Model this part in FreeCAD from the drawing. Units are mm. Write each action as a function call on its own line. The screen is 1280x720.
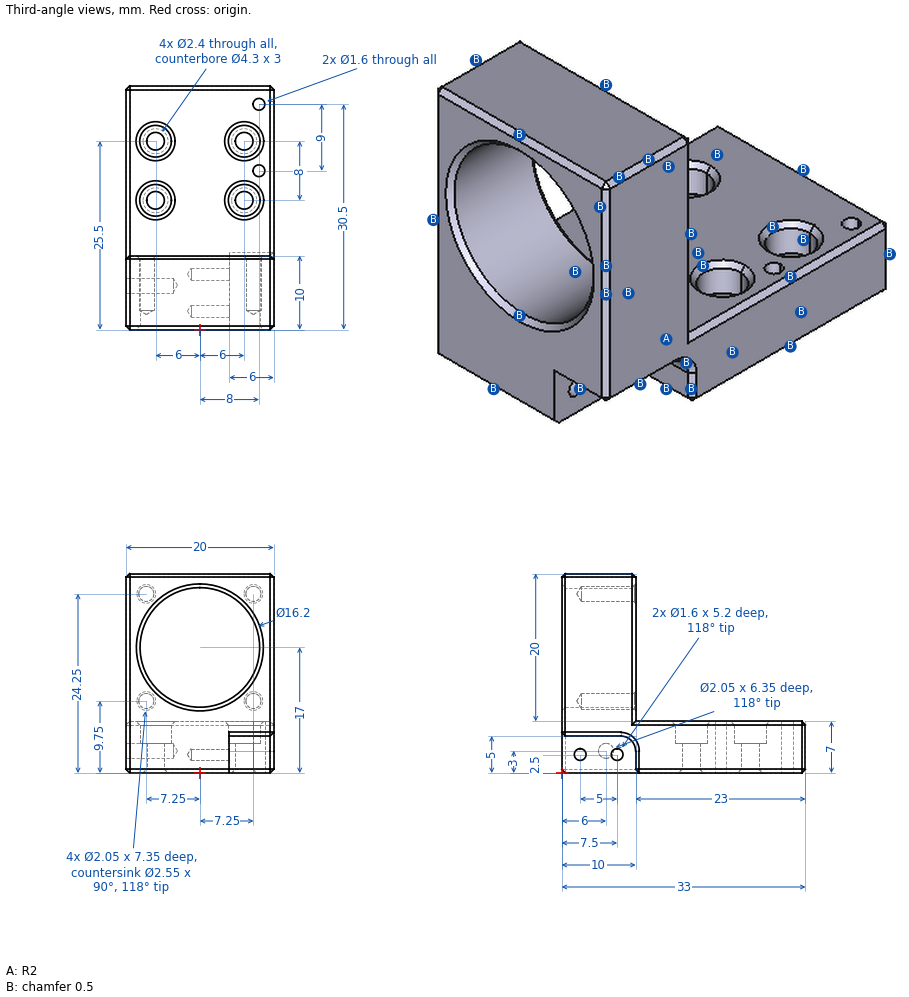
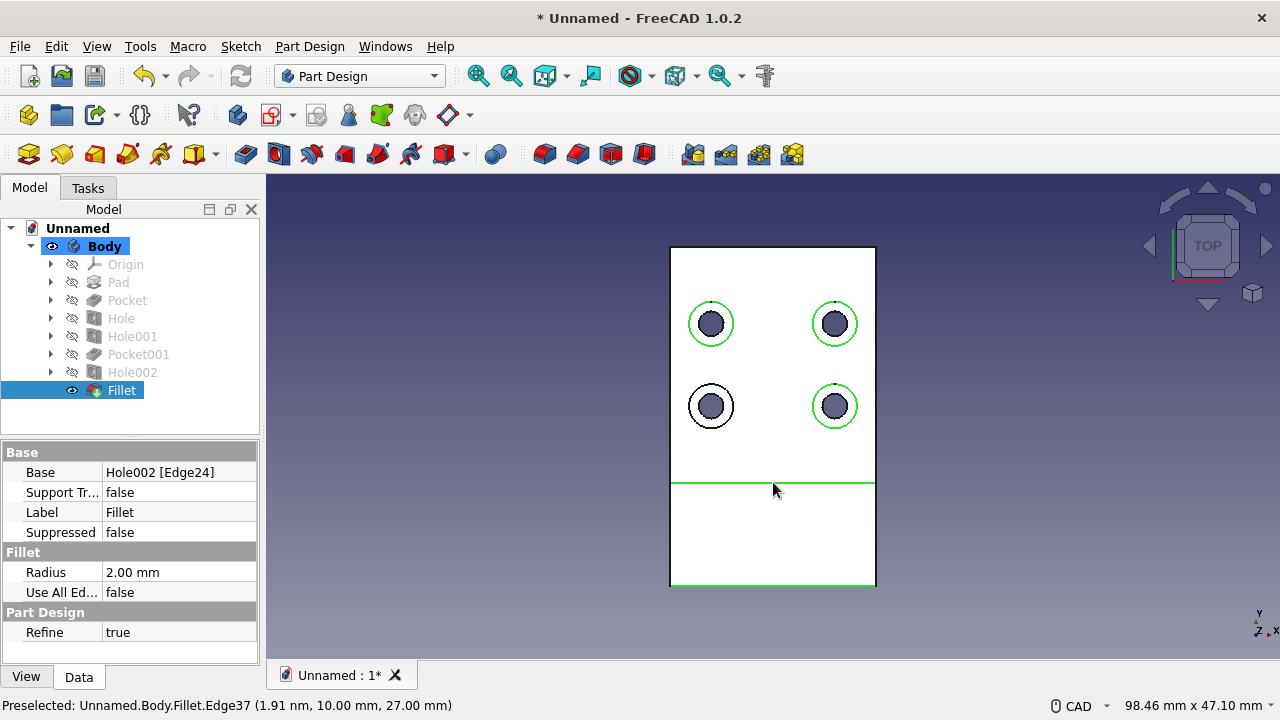
click(773, 246, ctrl)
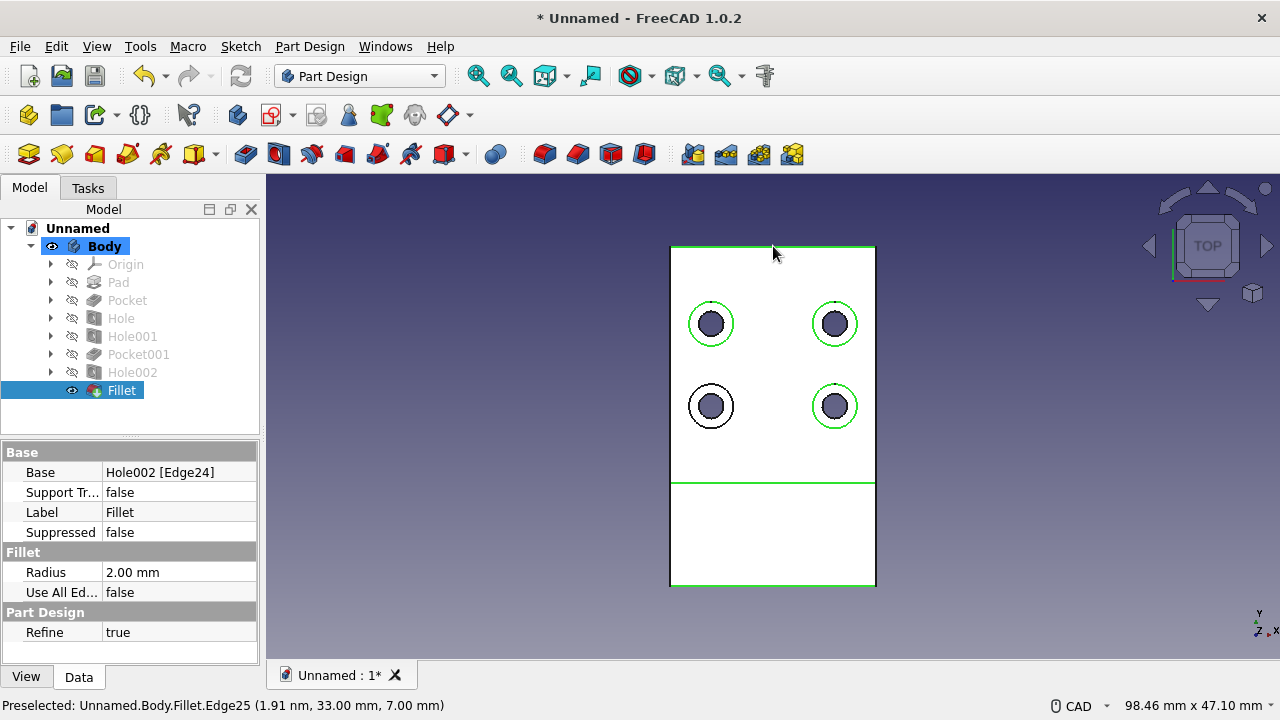
click(711, 427, ctrl)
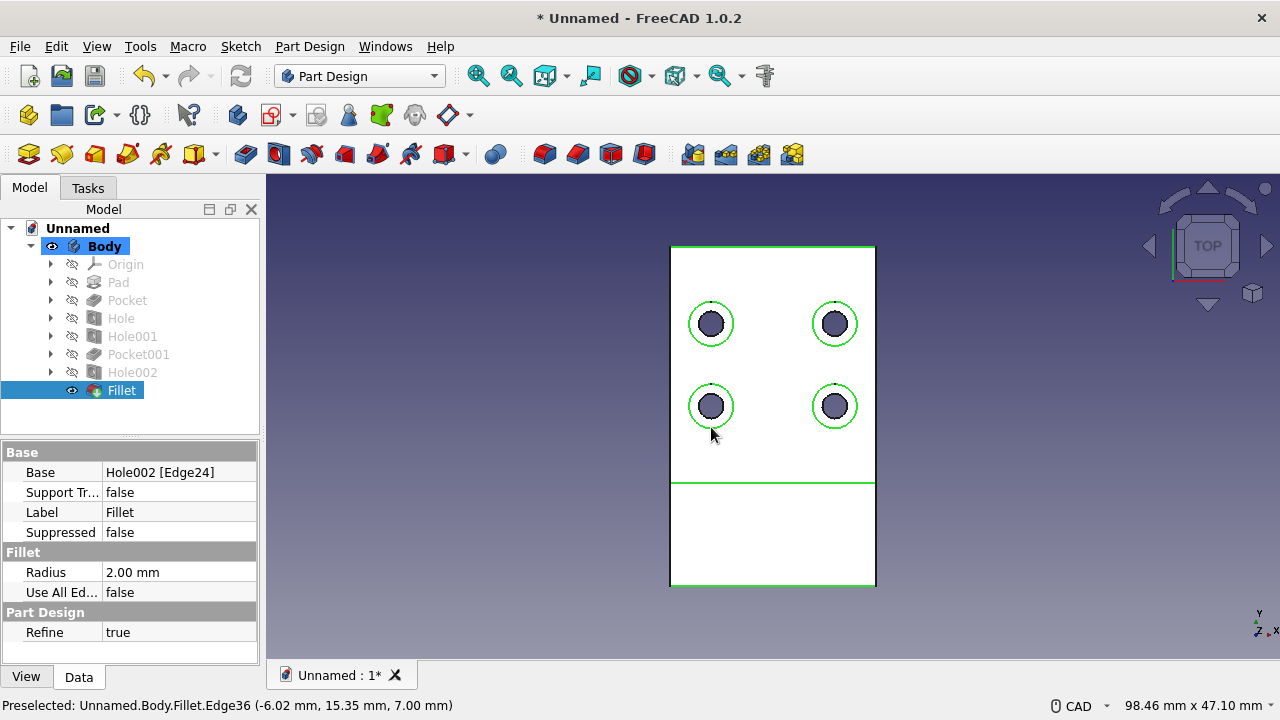
key(0)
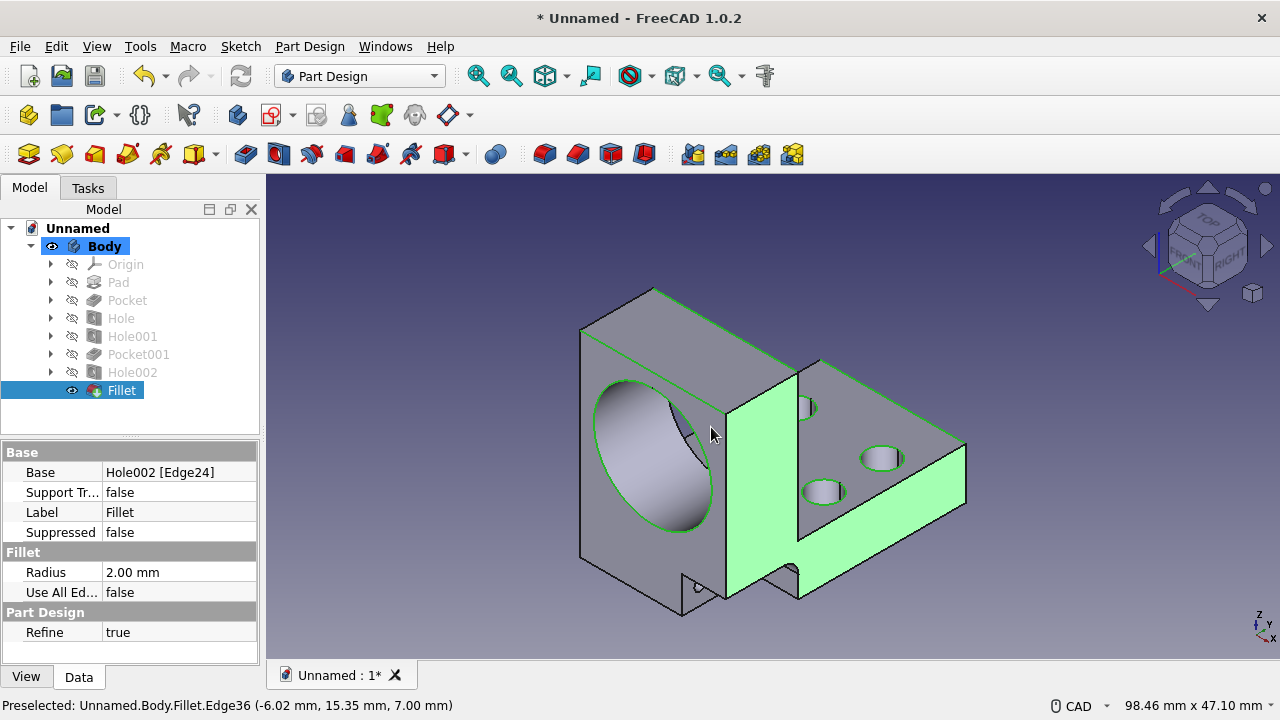
key(1)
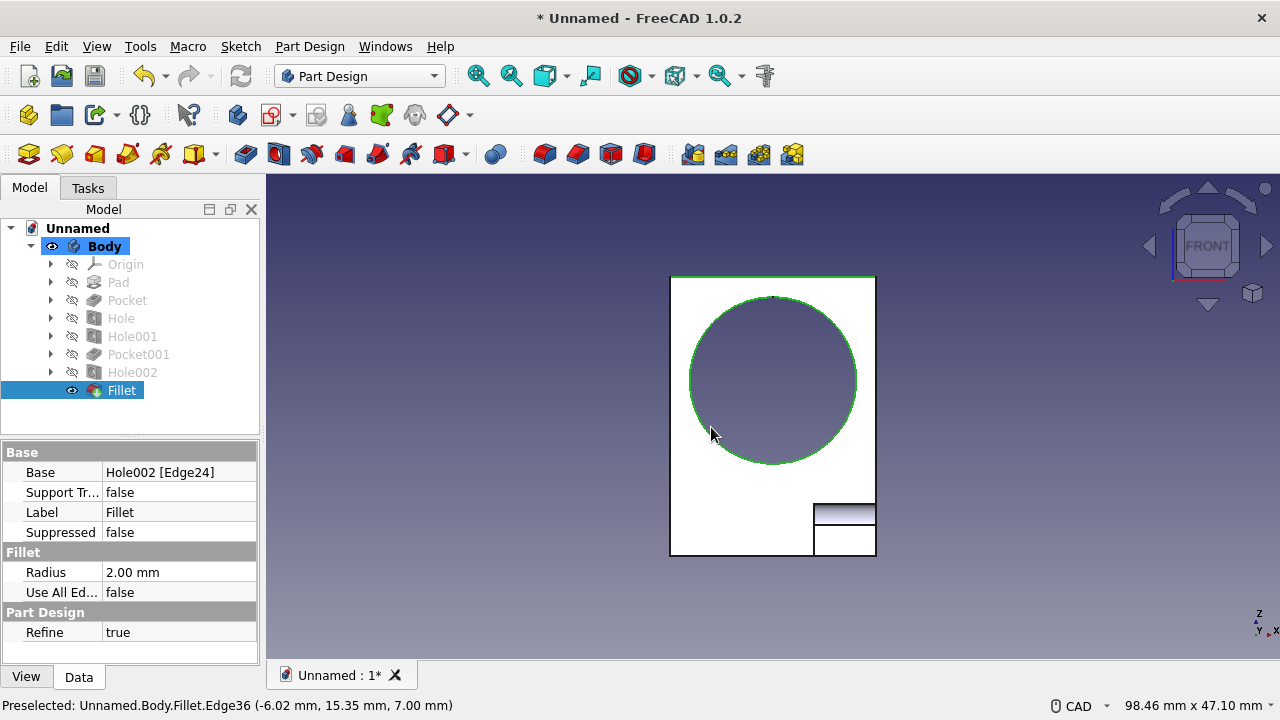
click(742, 555, ctrl)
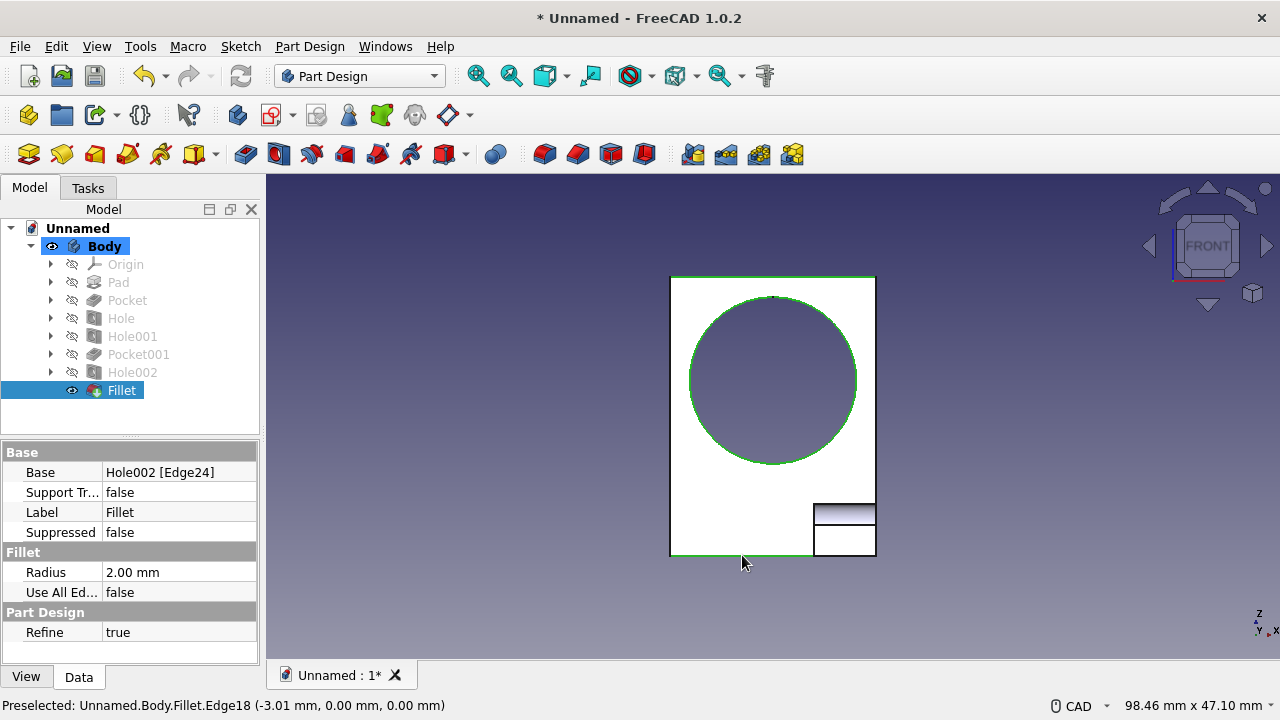
click(845, 555, ctrl)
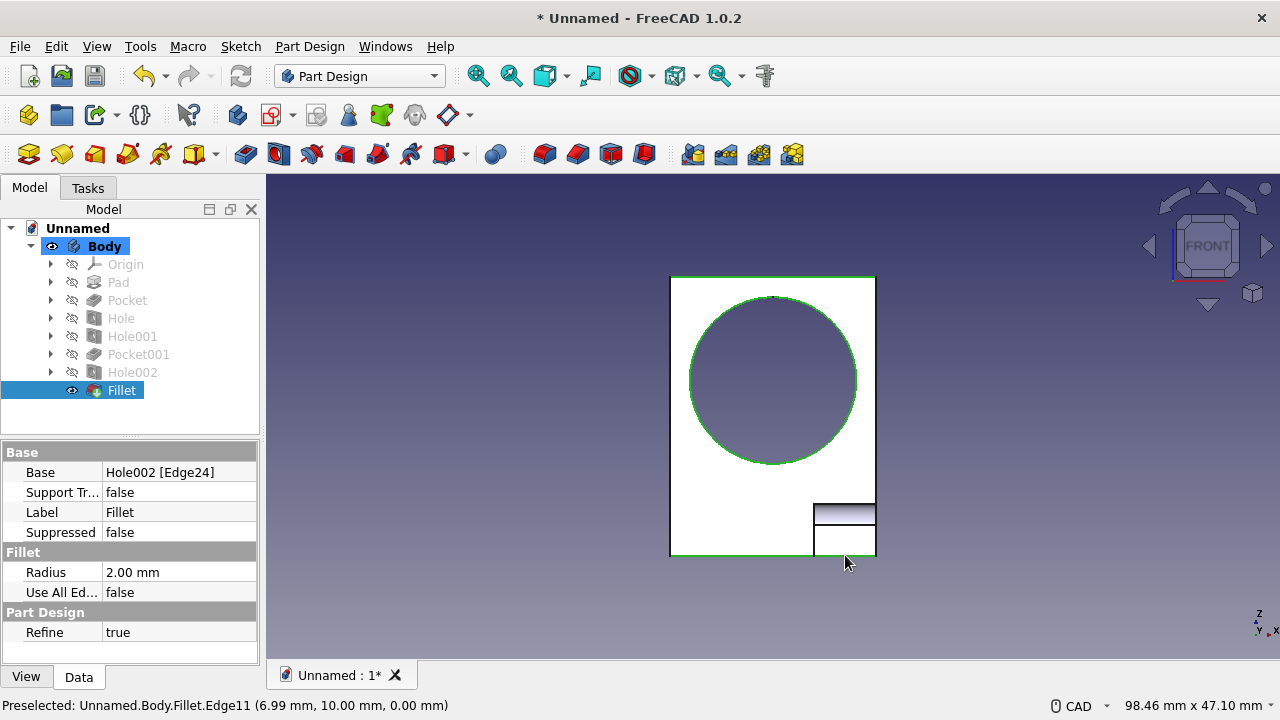
click(845, 503, ctrl)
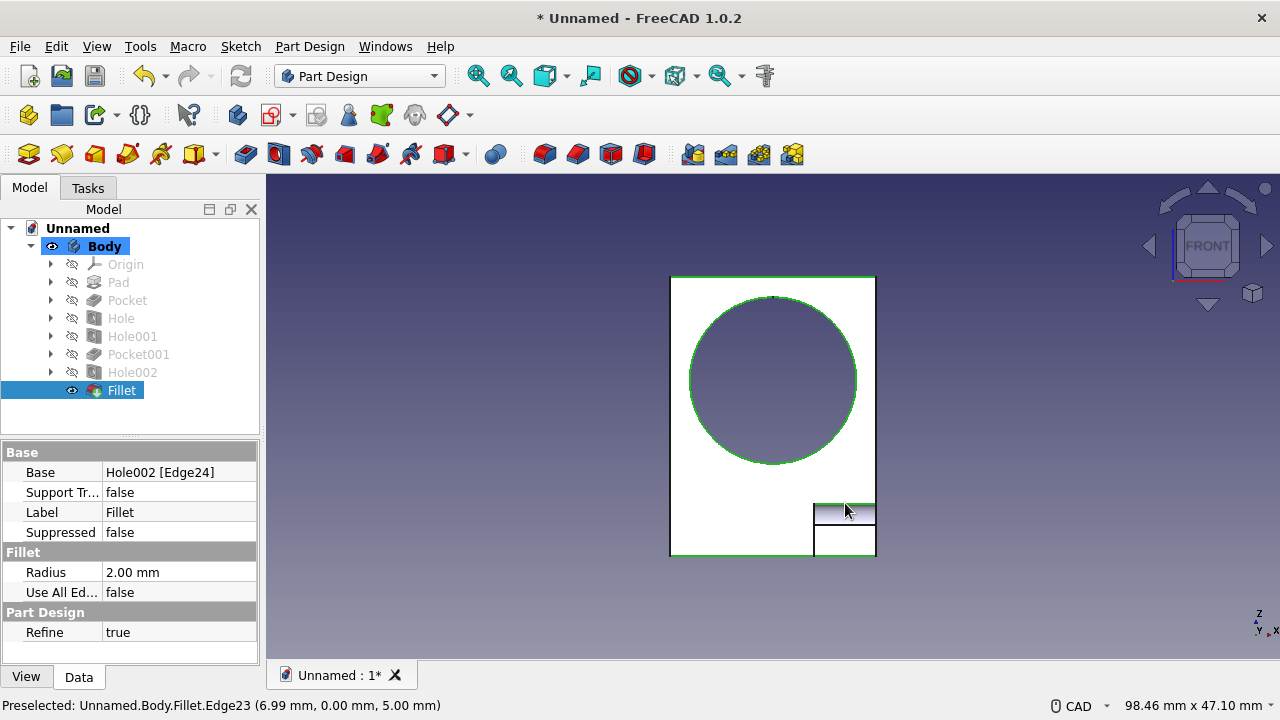
key(3)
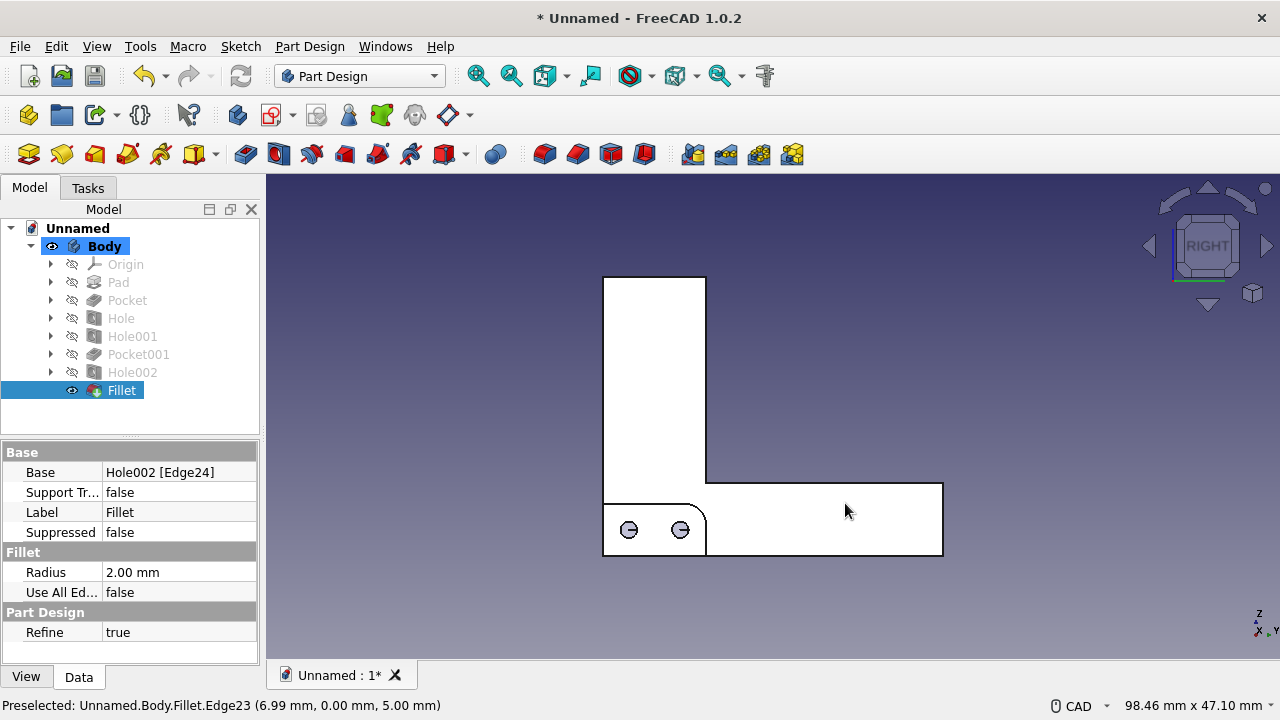
key(5)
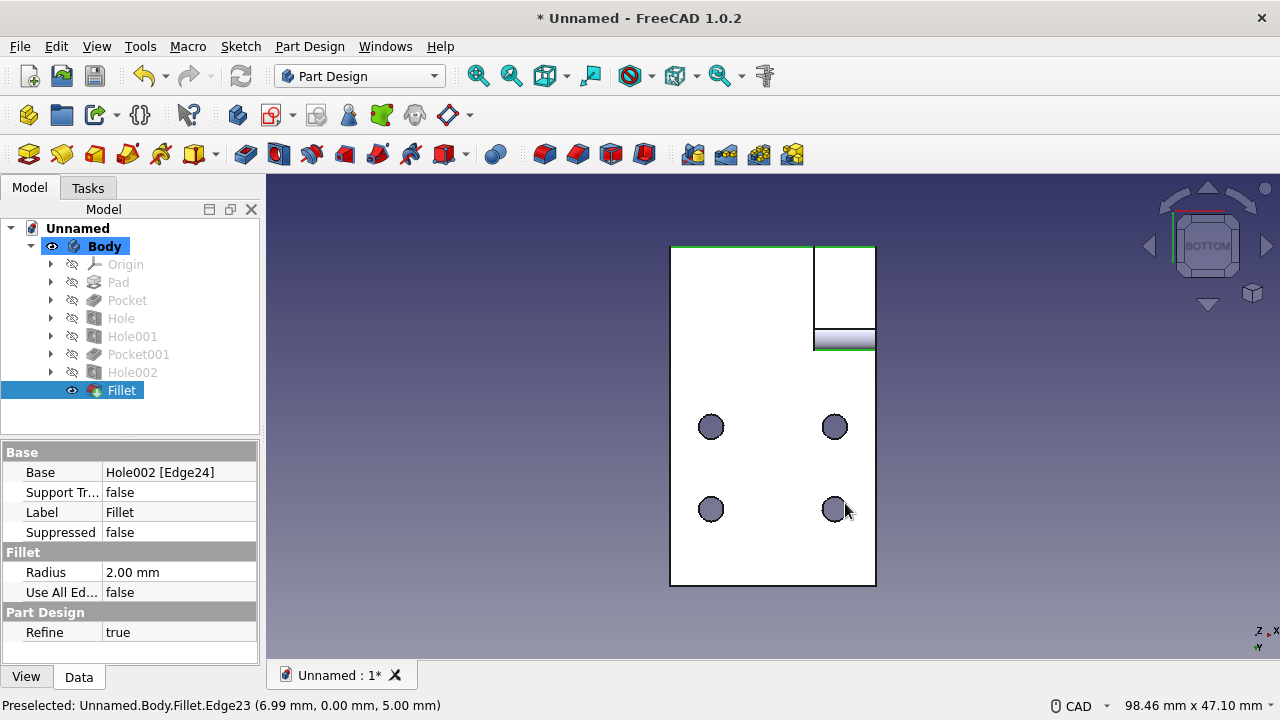
click(773, 585, ctrl)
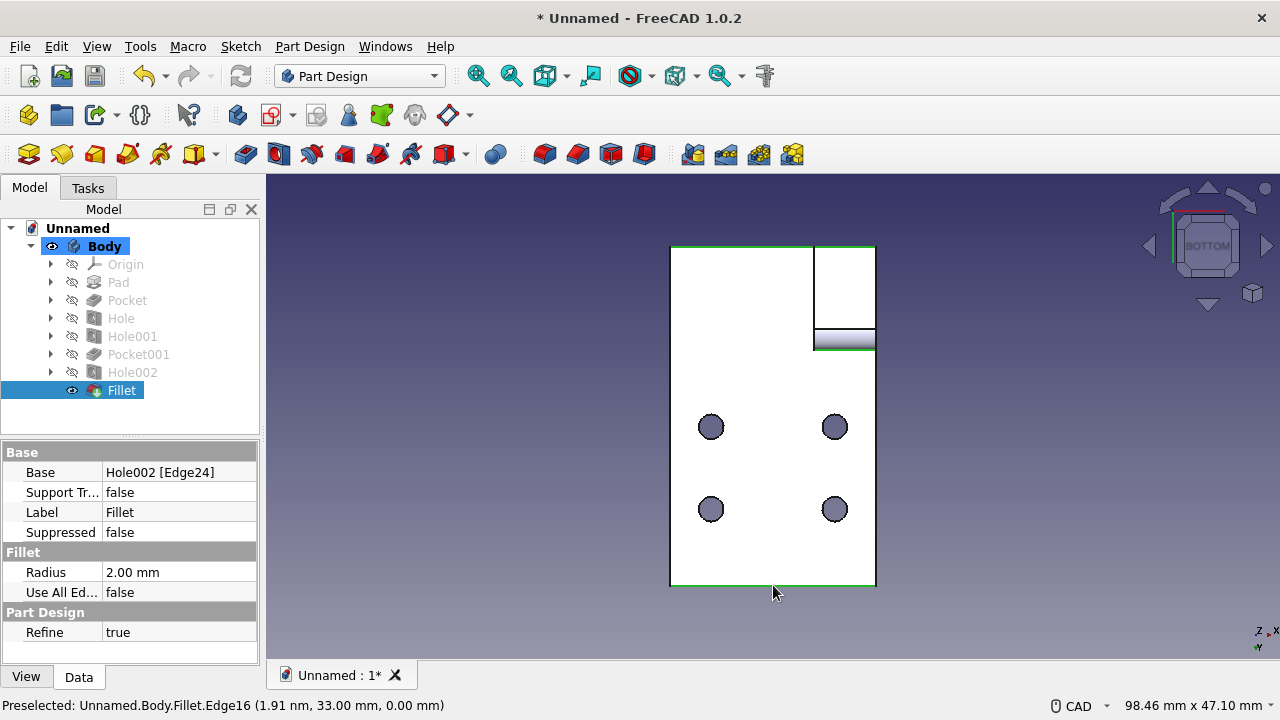
click(711, 413, ctrl)